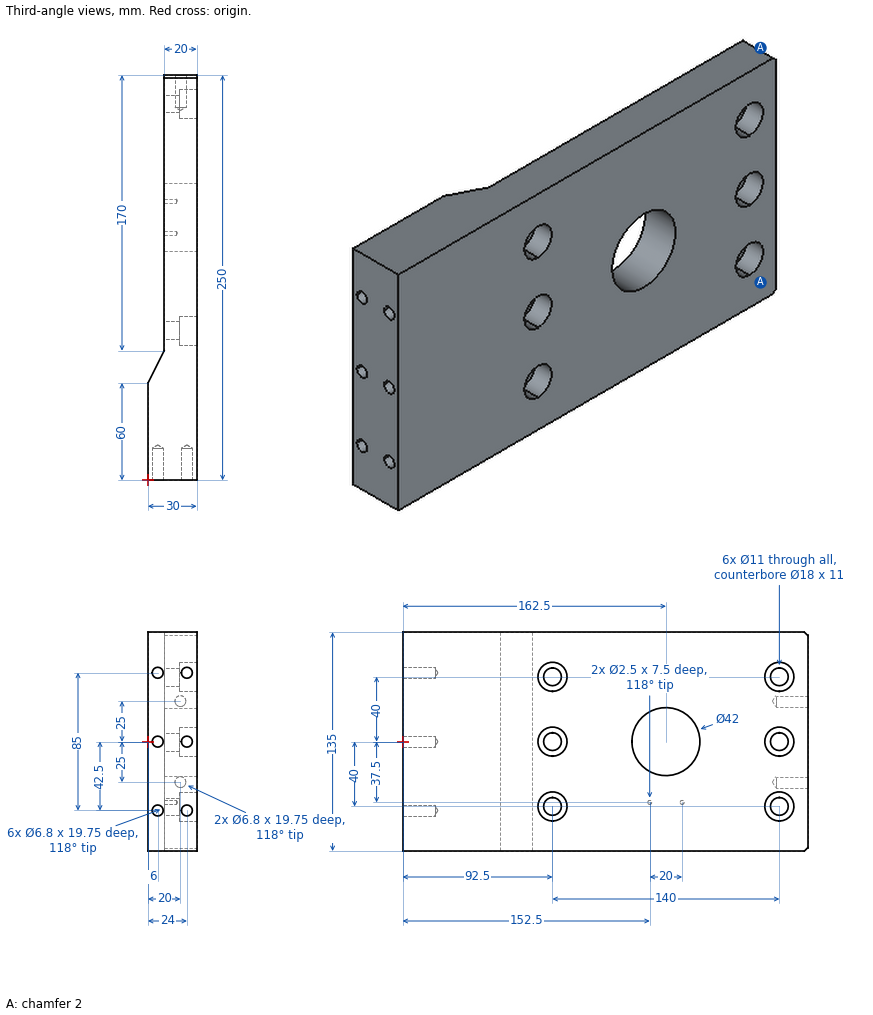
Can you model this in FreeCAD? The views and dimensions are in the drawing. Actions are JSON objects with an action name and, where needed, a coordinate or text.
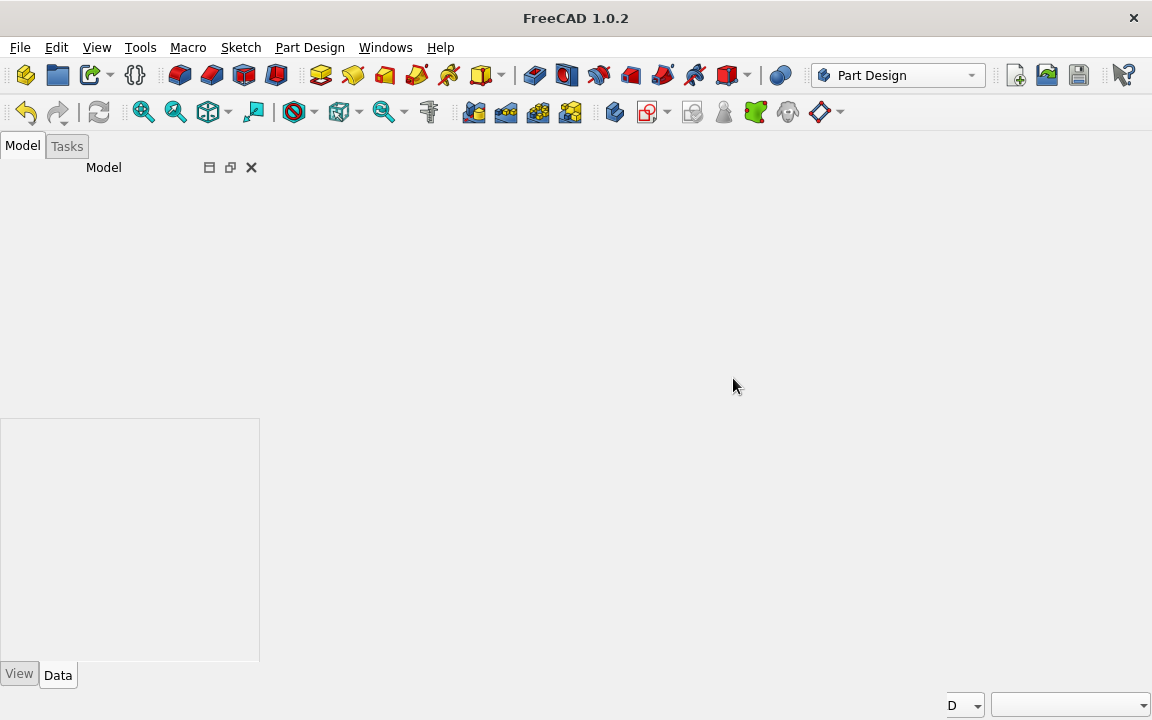
{"action": "left_click", "coordinate": [1016, 76]}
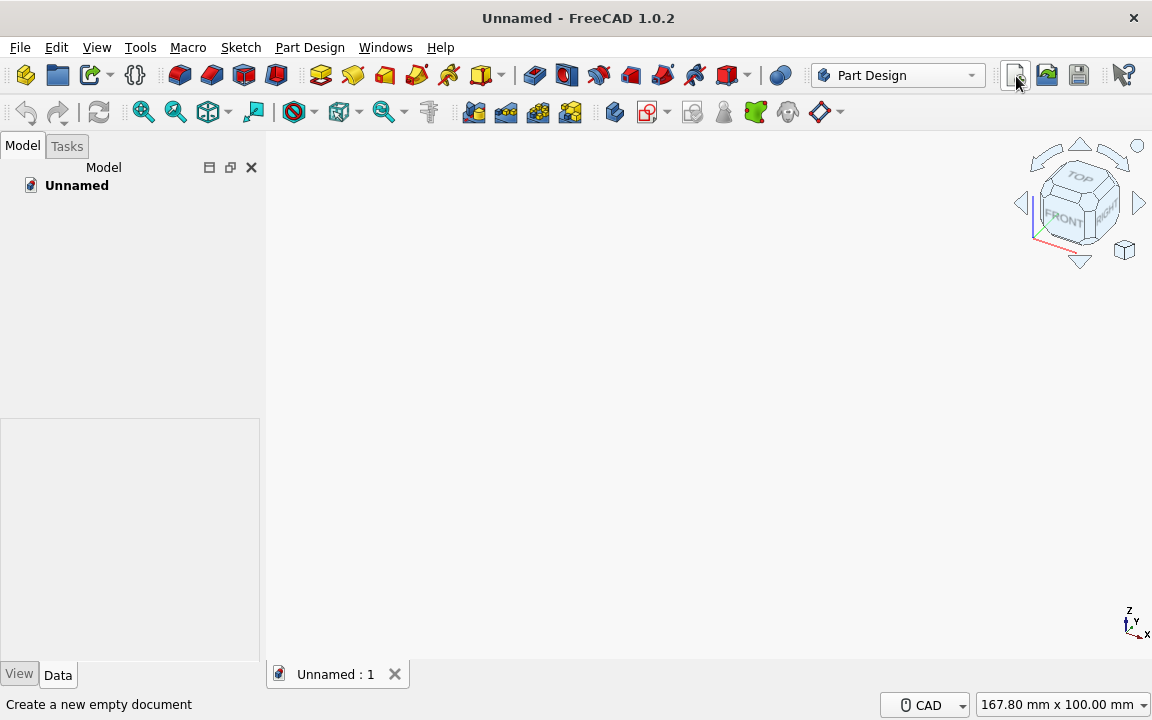
{"action": "left_click", "coordinate": [648, 112]}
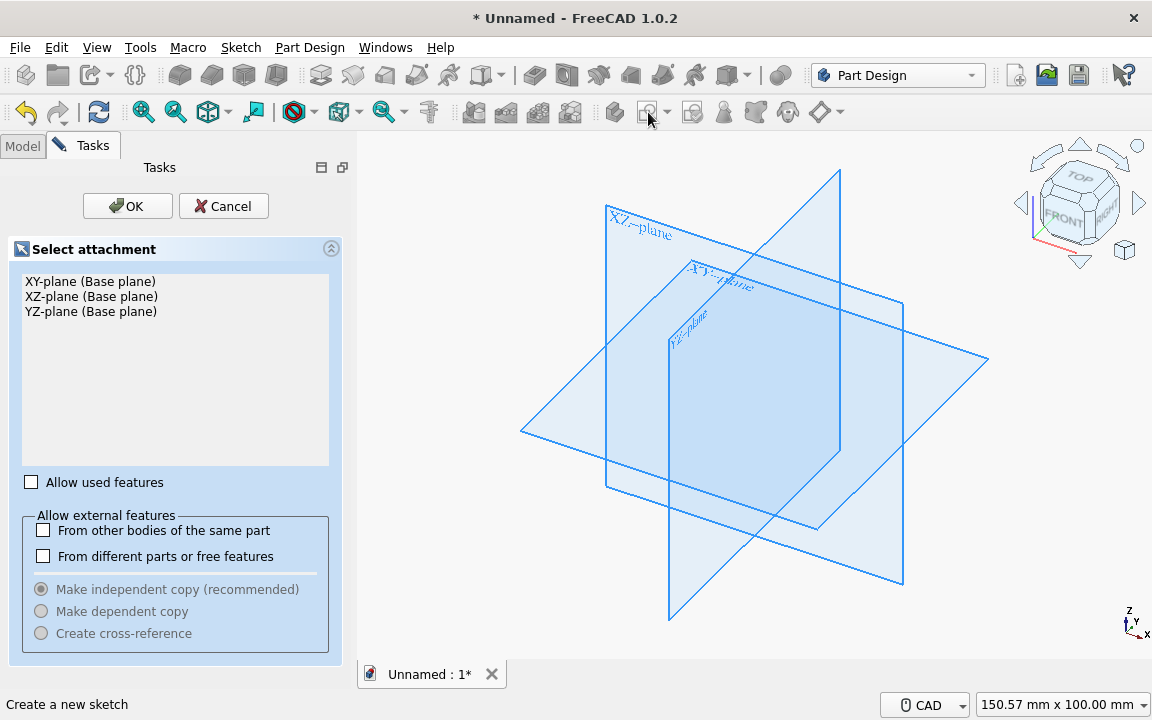
{"action": "left_click", "coordinate": [82, 282]}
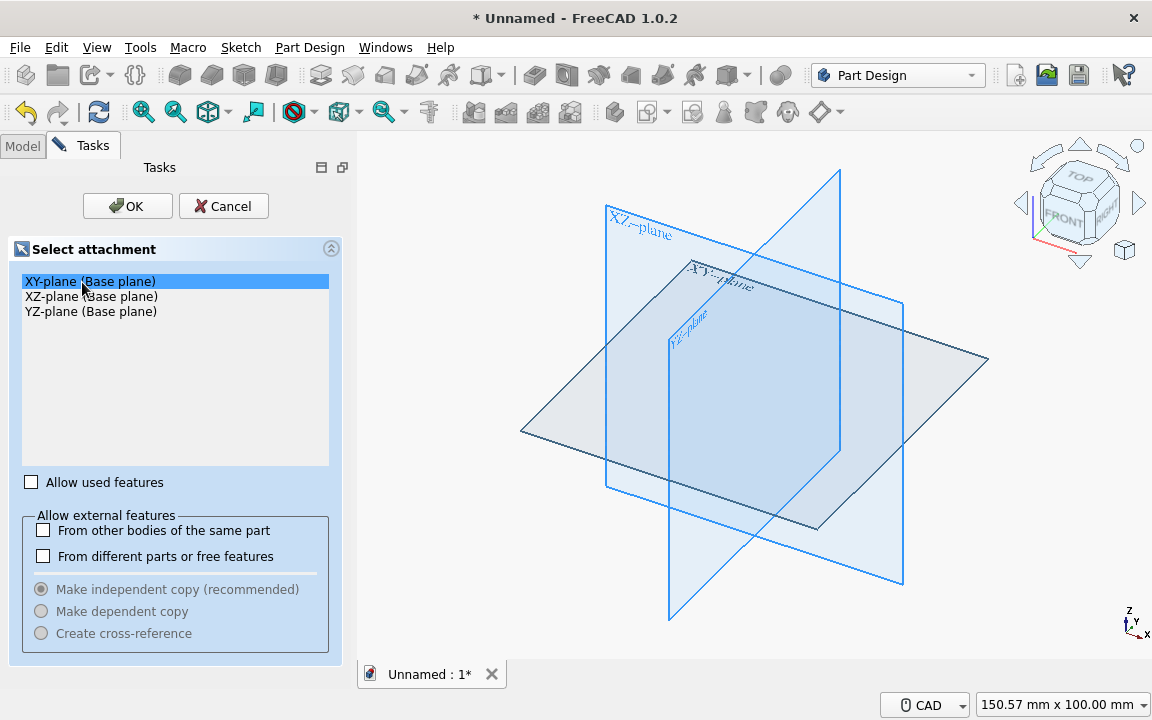
{"action": "left_click", "coordinate": [128, 206]}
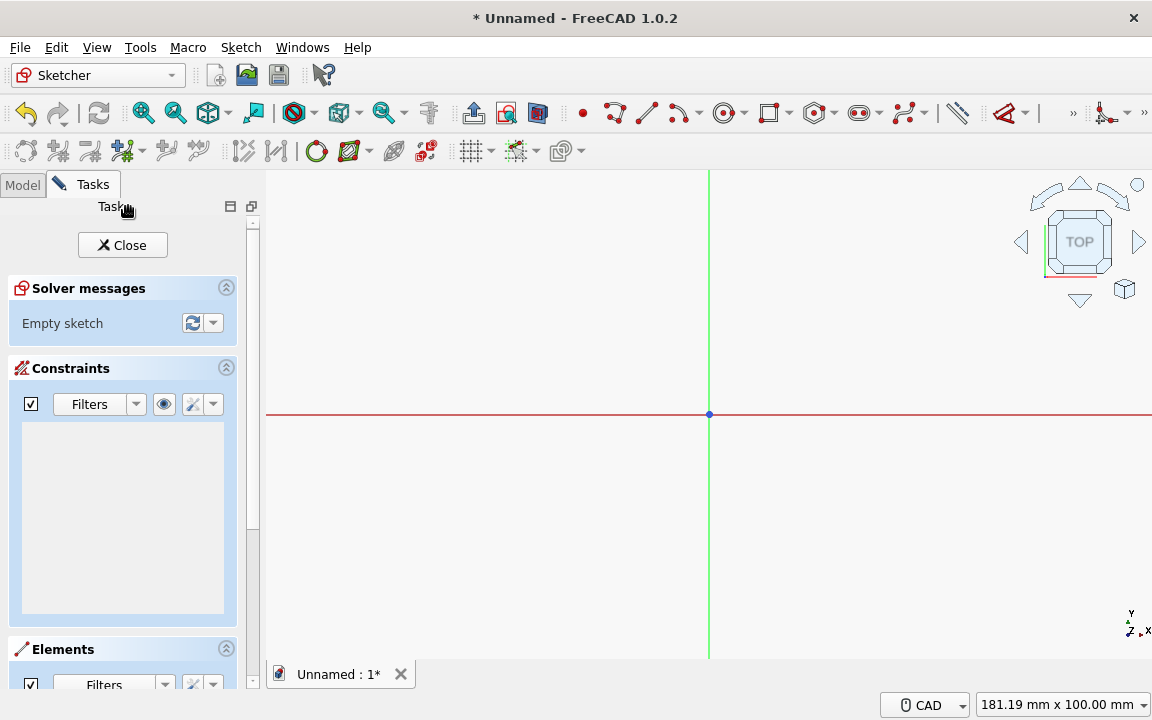
{"action": "scroll", "coordinate": [594, 615], "scroll_direction": "down", "scroll_amount": 7}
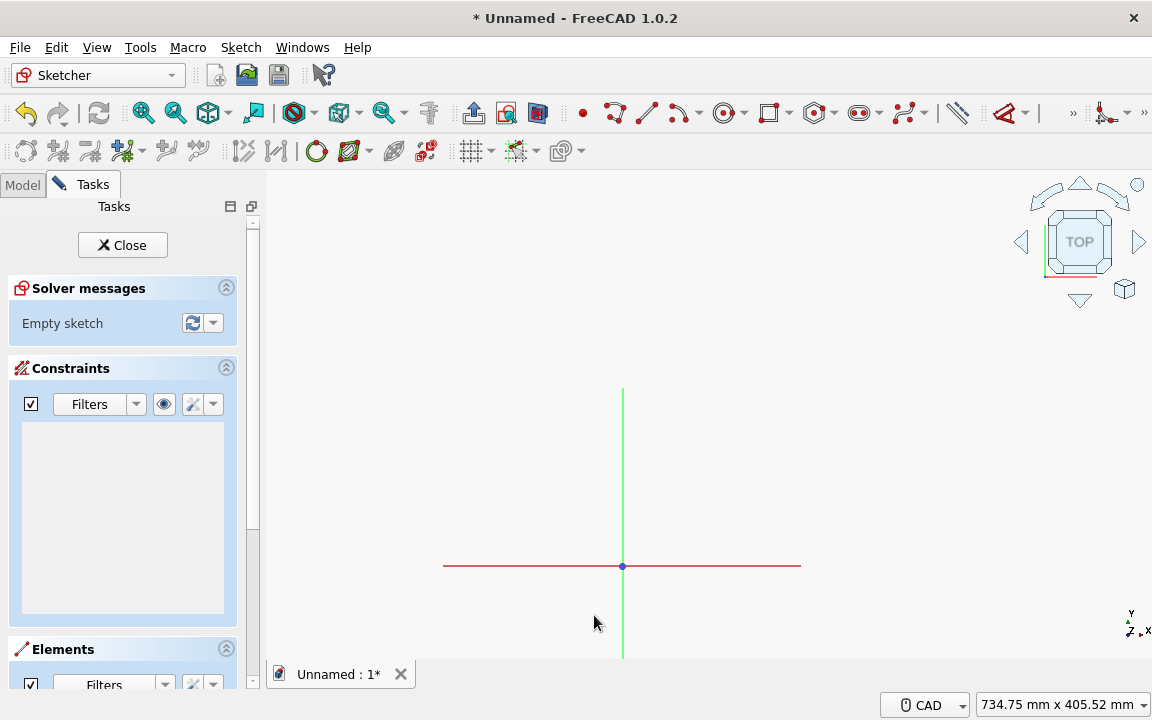
{"action": "left_click", "coordinate": [616, 114]}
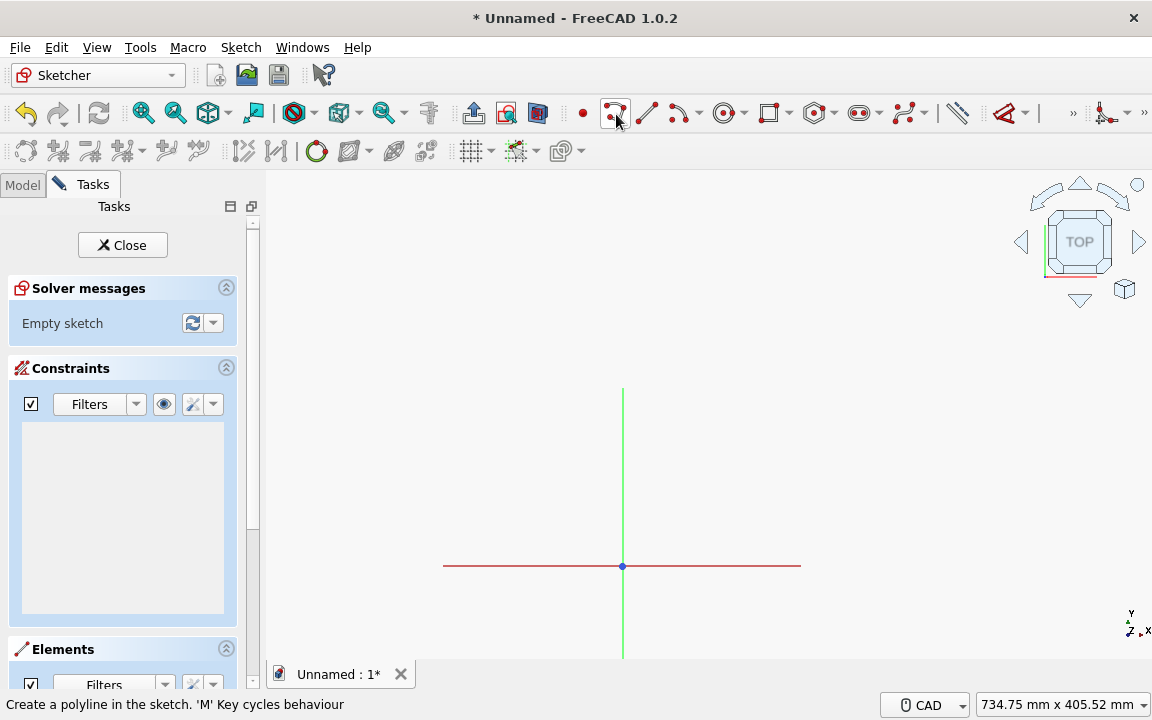
{"action": "left_click", "coordinate": [623, 566]}
{"action": "left_click", "coordinate": [659, 557]}
{"action": "left_click", "coordinate": [659, 265]}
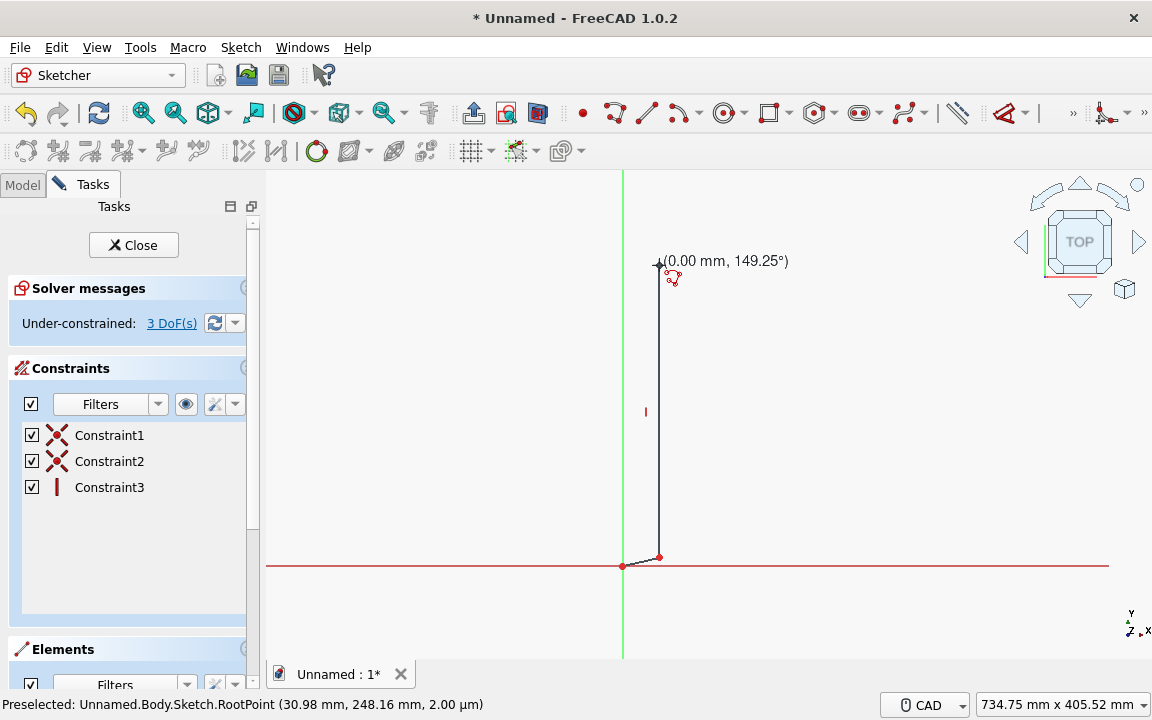
{"action": "scroll", "coordinate": [635, 265], "scroll_direction": "up", "scroll_amount": 2}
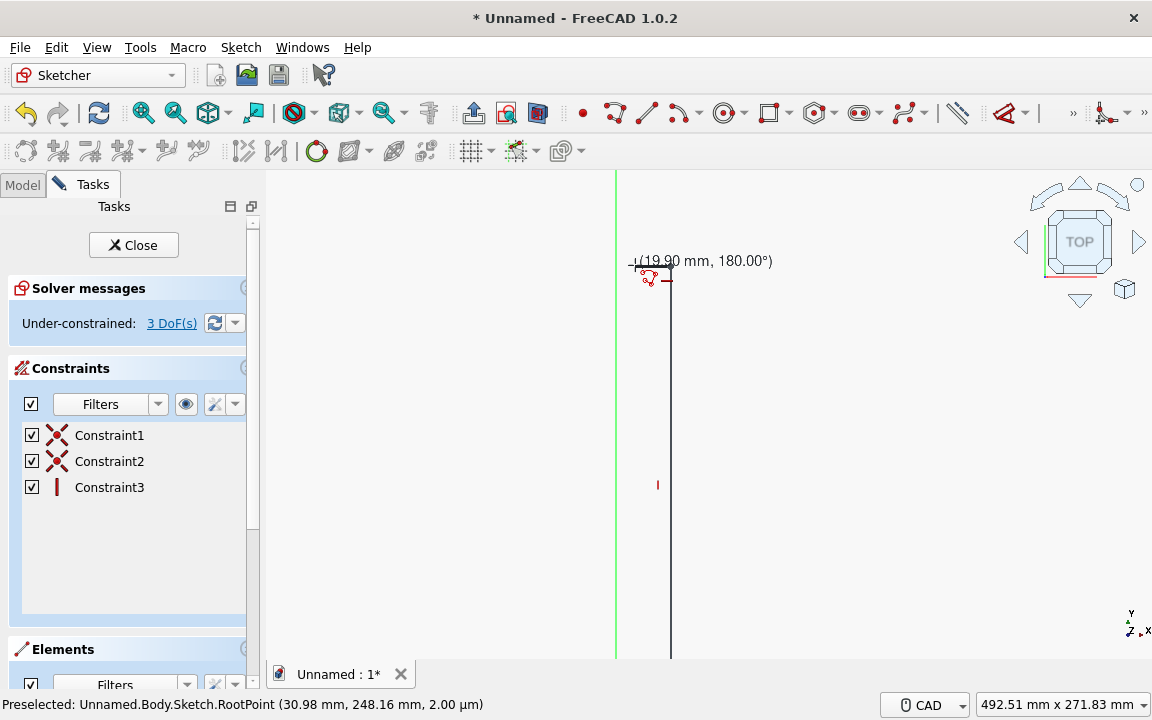
{"action": "left_click", "coordinate": [634, 265]}
{"action": "left_click", "coordinate": [634, 570]}
{"action": "left_click", "coordinate": [625, 606]}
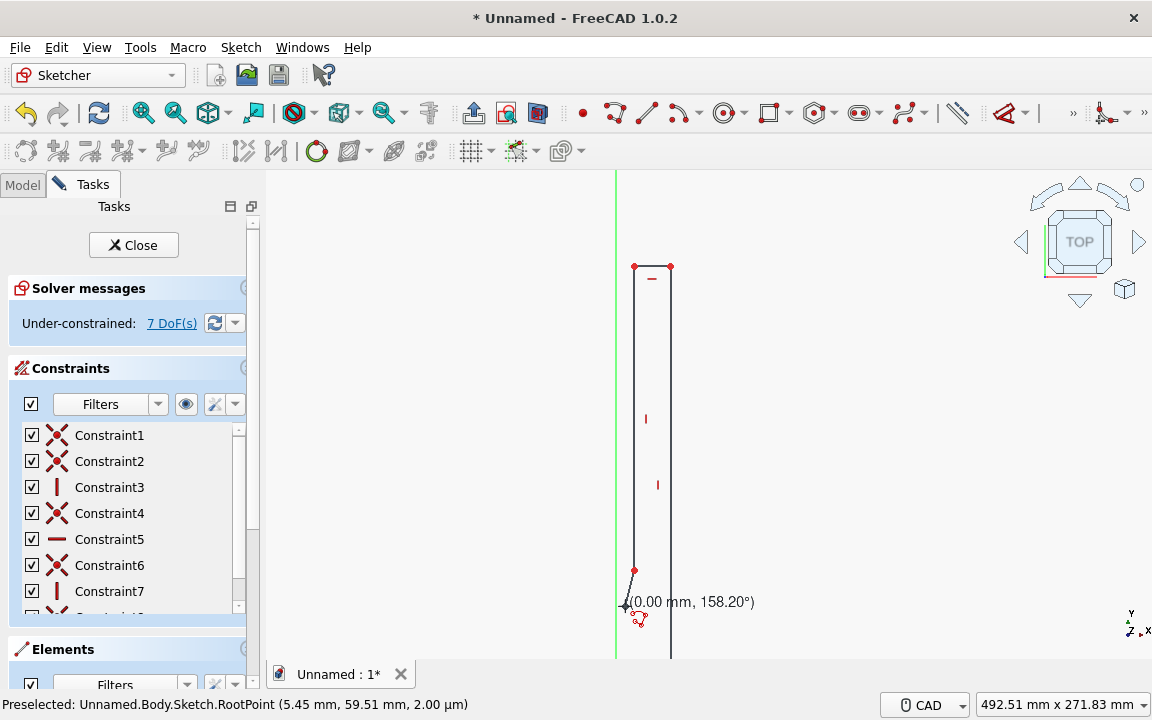
{"action": "scroll", "coordinate": [635, 262], "scroll_direction": "down", "scroll_amount": 2}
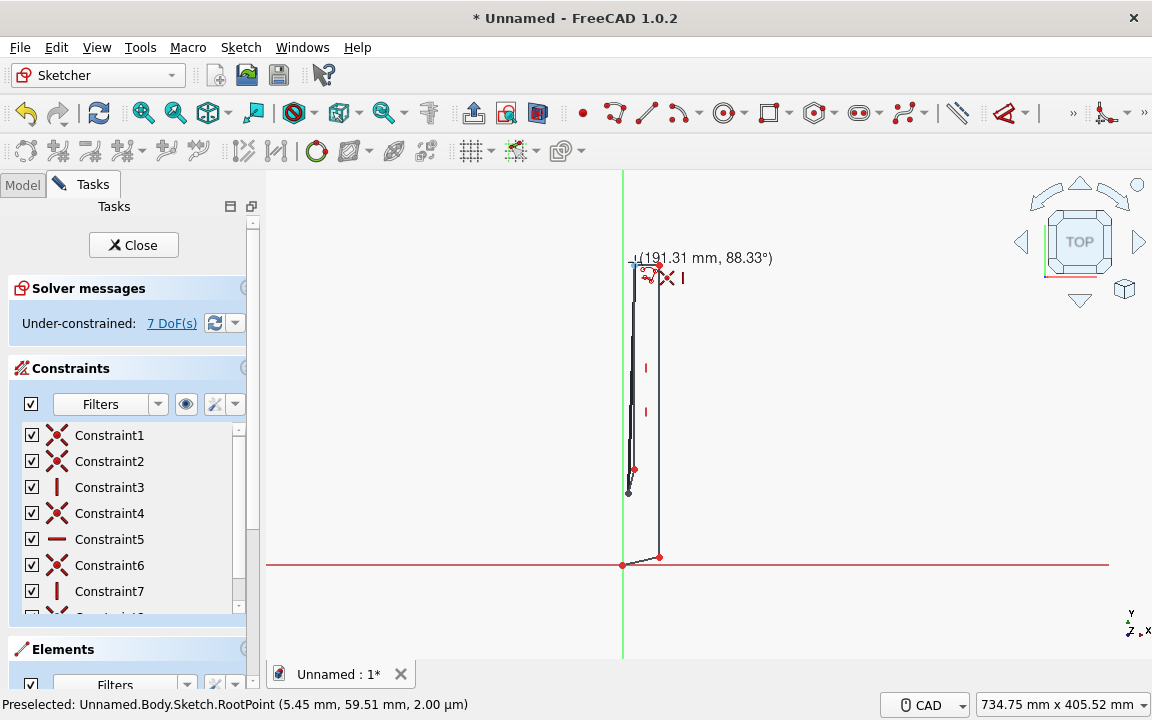
{"action": "left_click", "coordinate": [623, 565]}
{"action": "key", "text": "Escape"}
{"action": "key", "text": "Escape"}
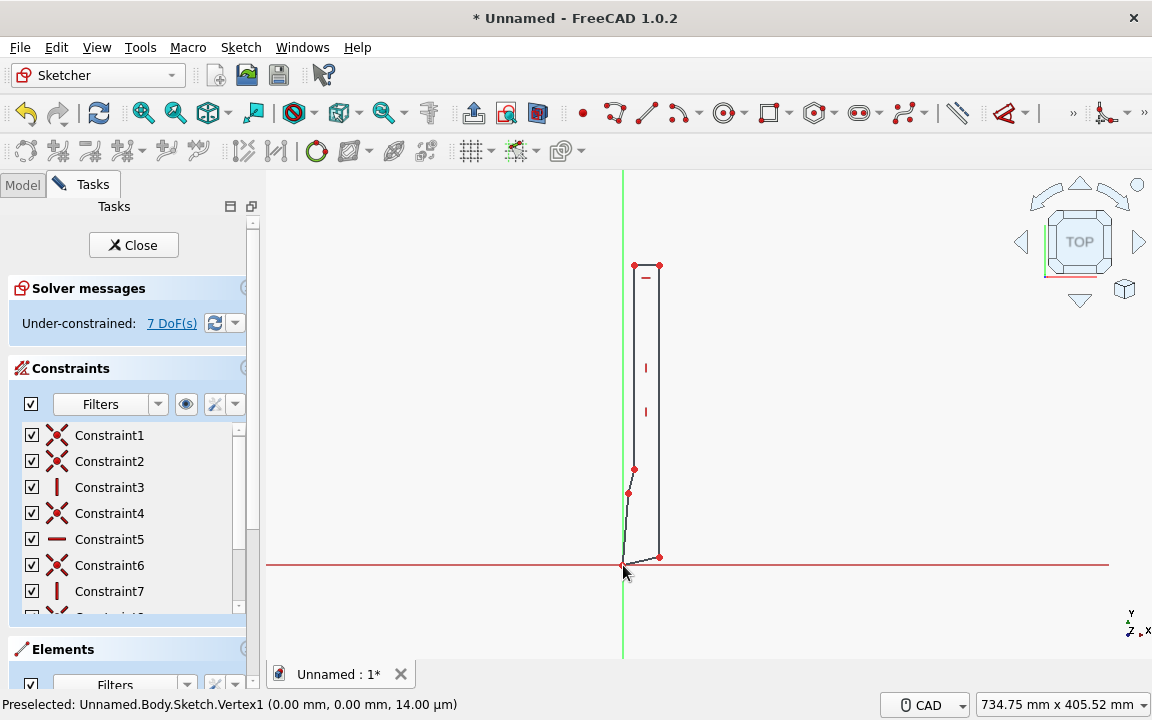
{"action": "scroll", "coordinate": [634, 563], "scroll_direction": "up", "scroll_amount": 2}